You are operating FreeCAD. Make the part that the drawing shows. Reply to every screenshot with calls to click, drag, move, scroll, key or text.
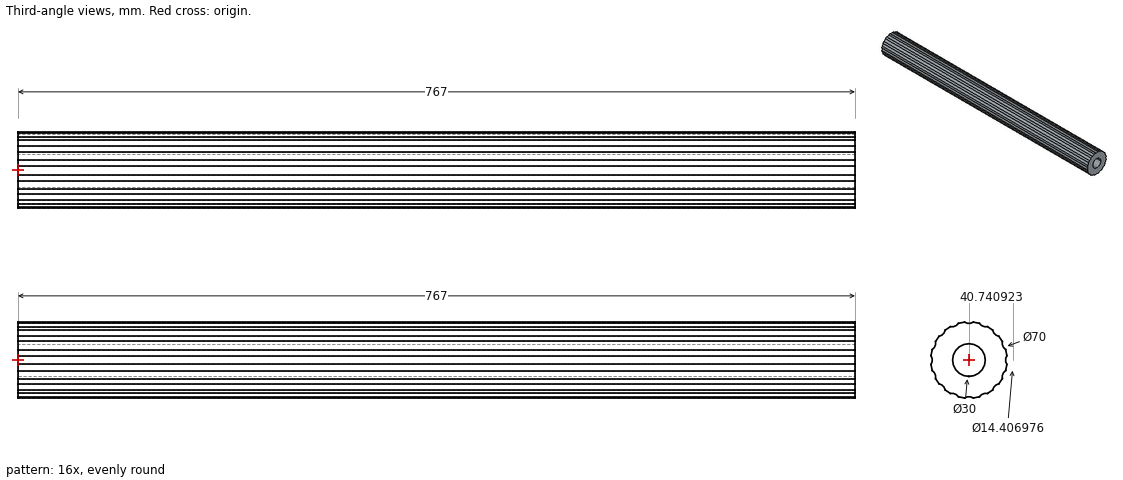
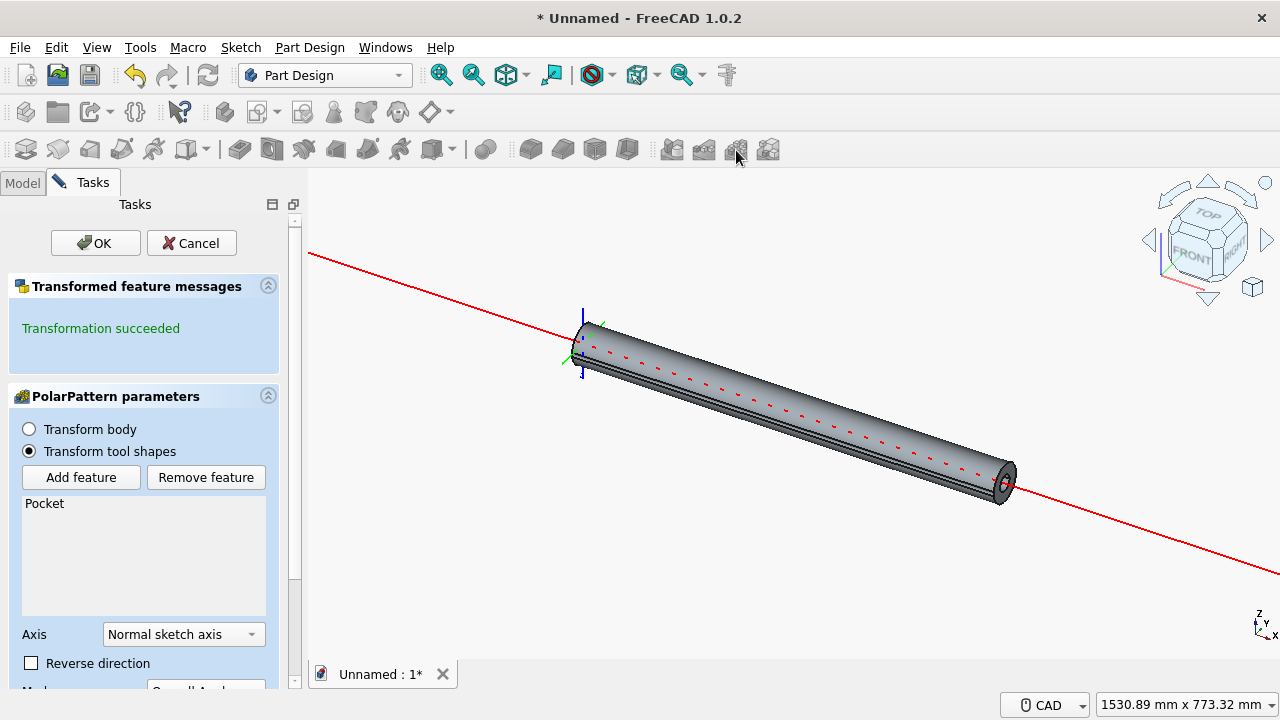
click(184, 634)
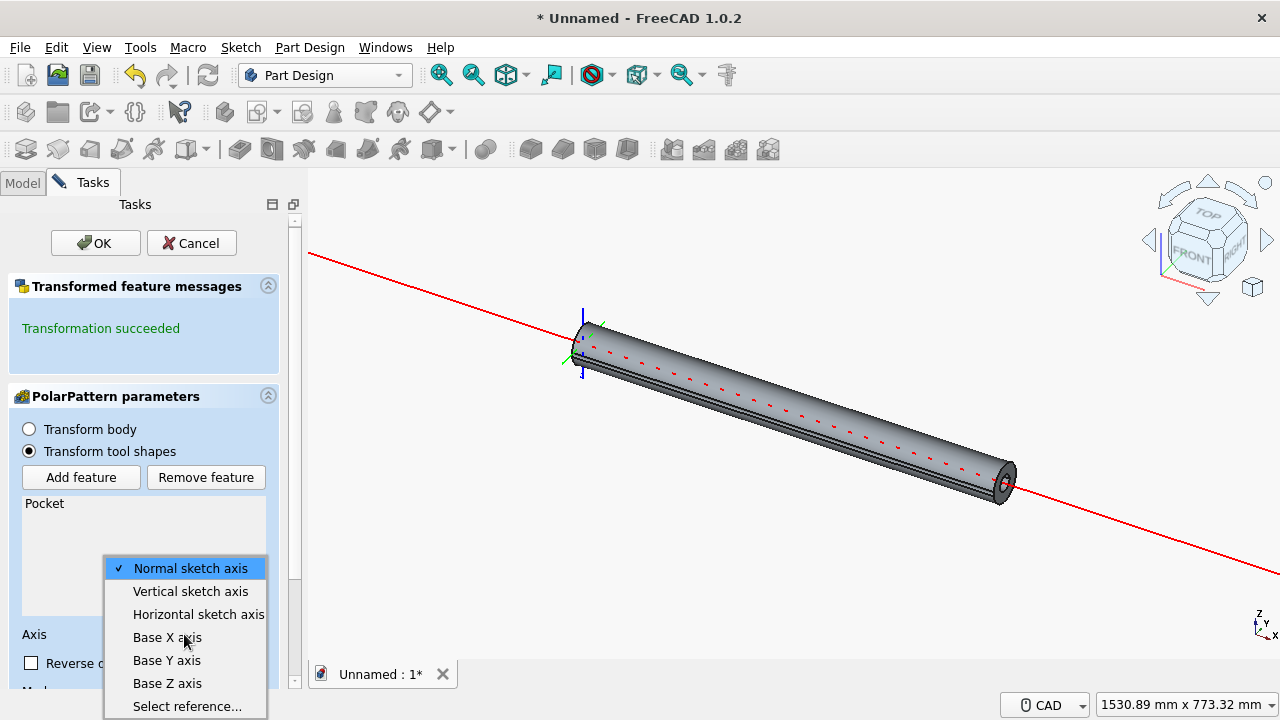
click(184, 638)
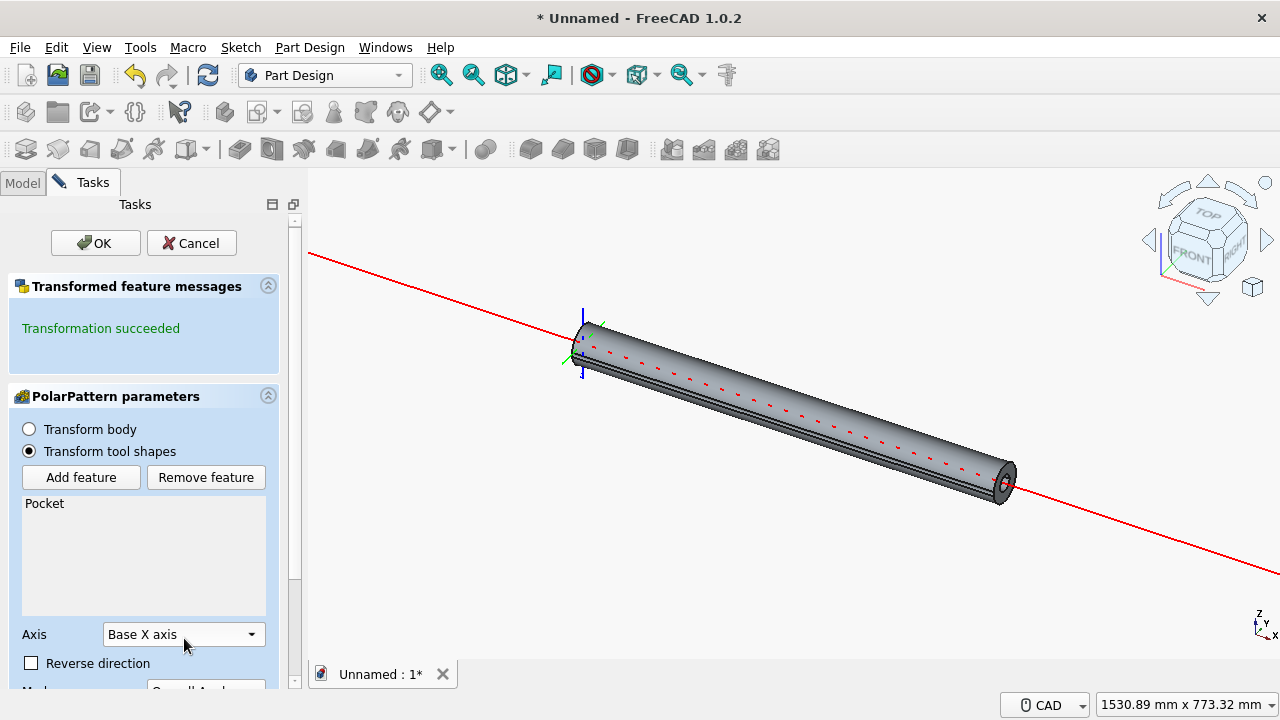
scroll(295, 451, down, 3)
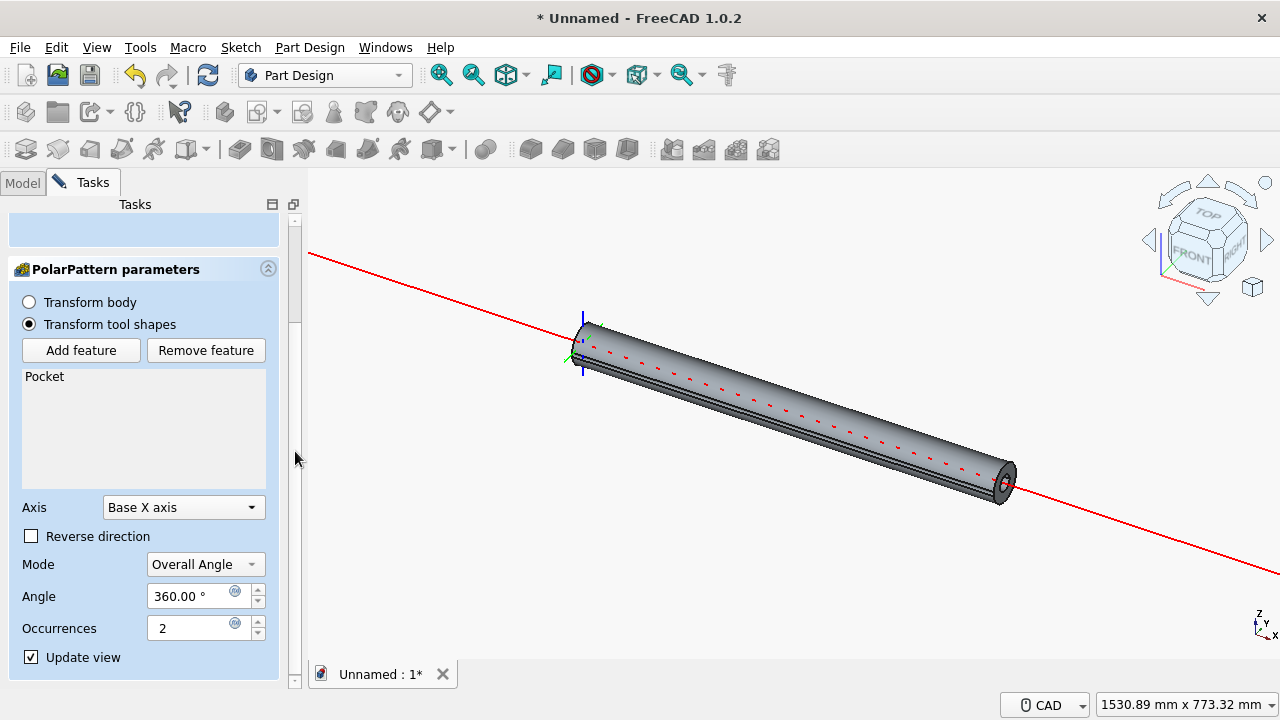
triple_click(198, 628)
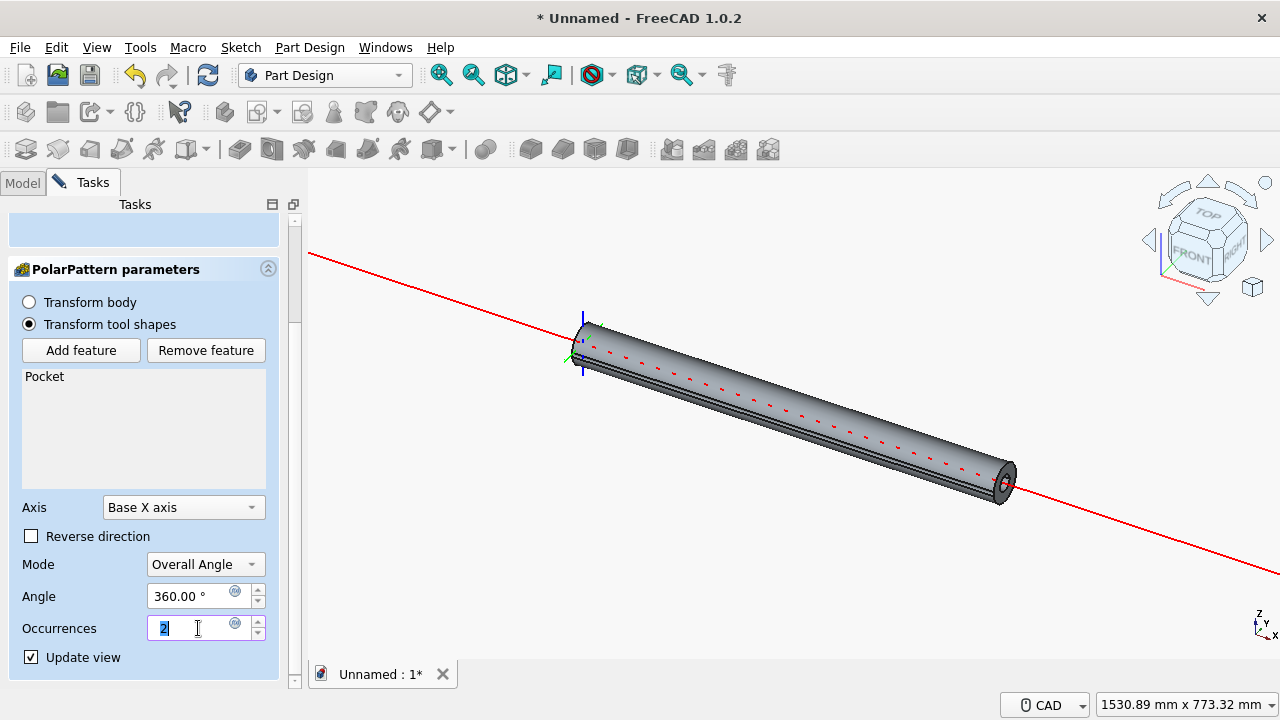
text(16)
key(Tab)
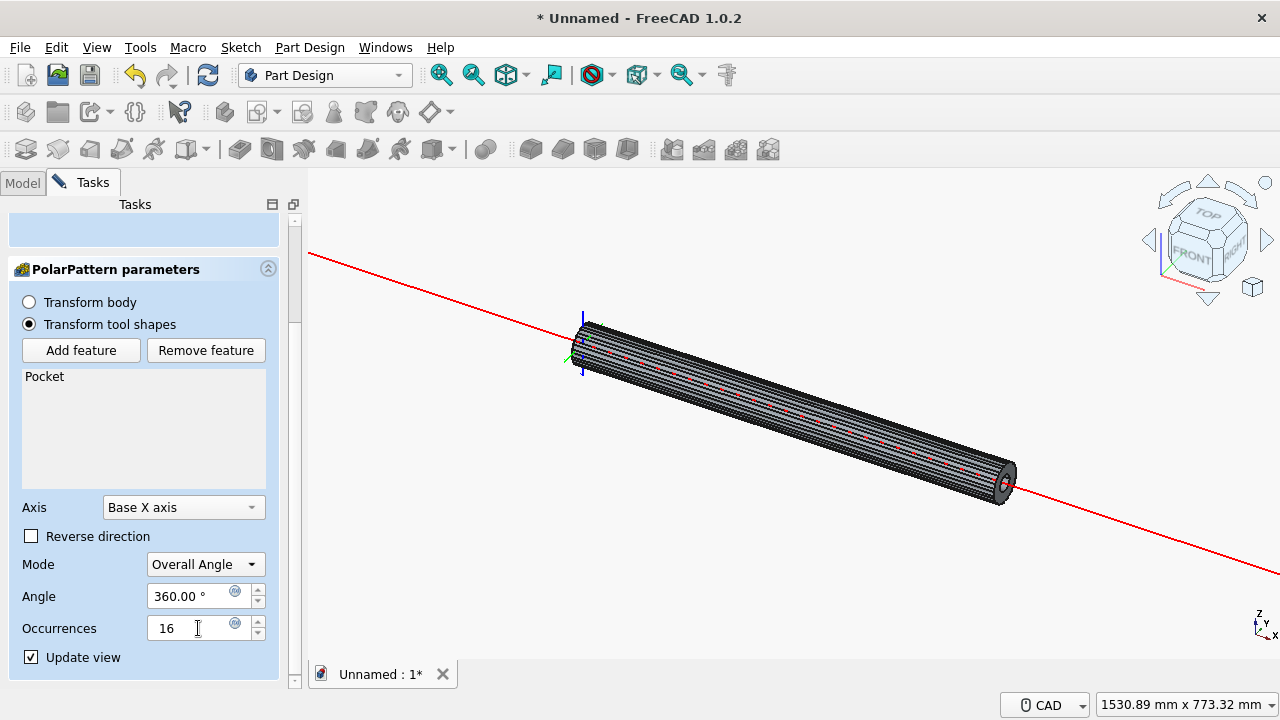
scroll(295, 451, up, 3)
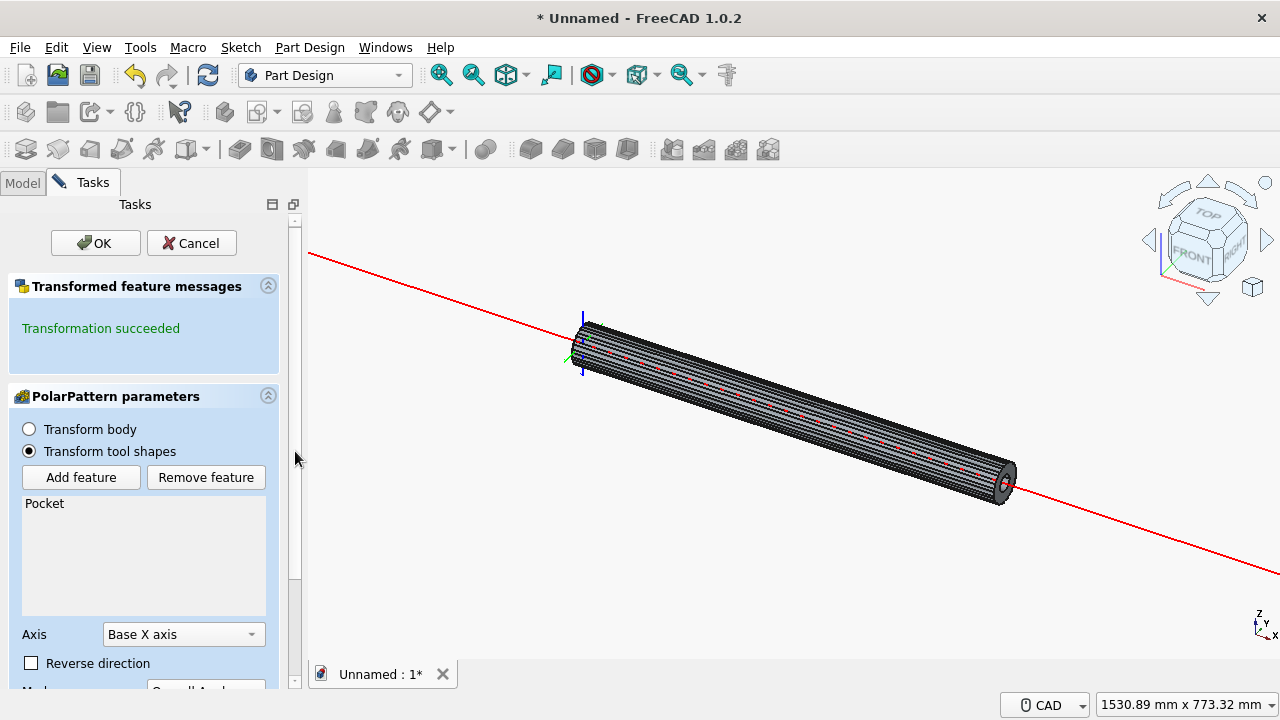
click(96, 243)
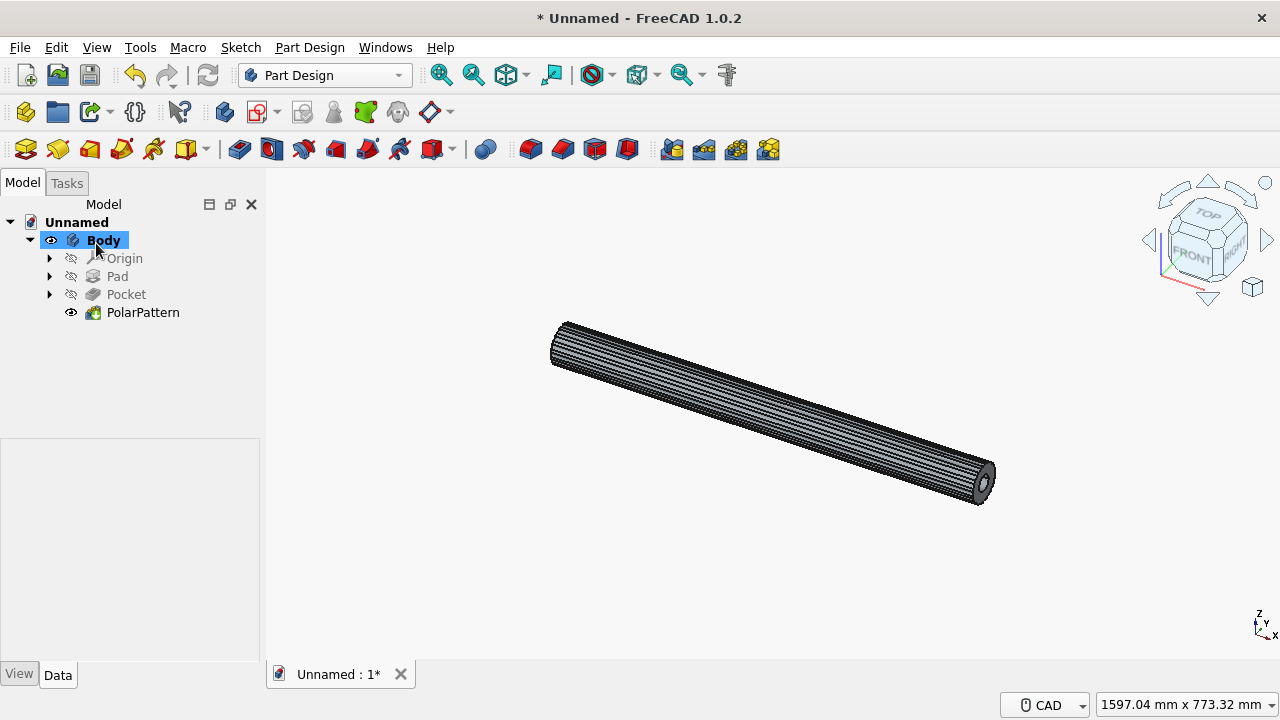
key(0)